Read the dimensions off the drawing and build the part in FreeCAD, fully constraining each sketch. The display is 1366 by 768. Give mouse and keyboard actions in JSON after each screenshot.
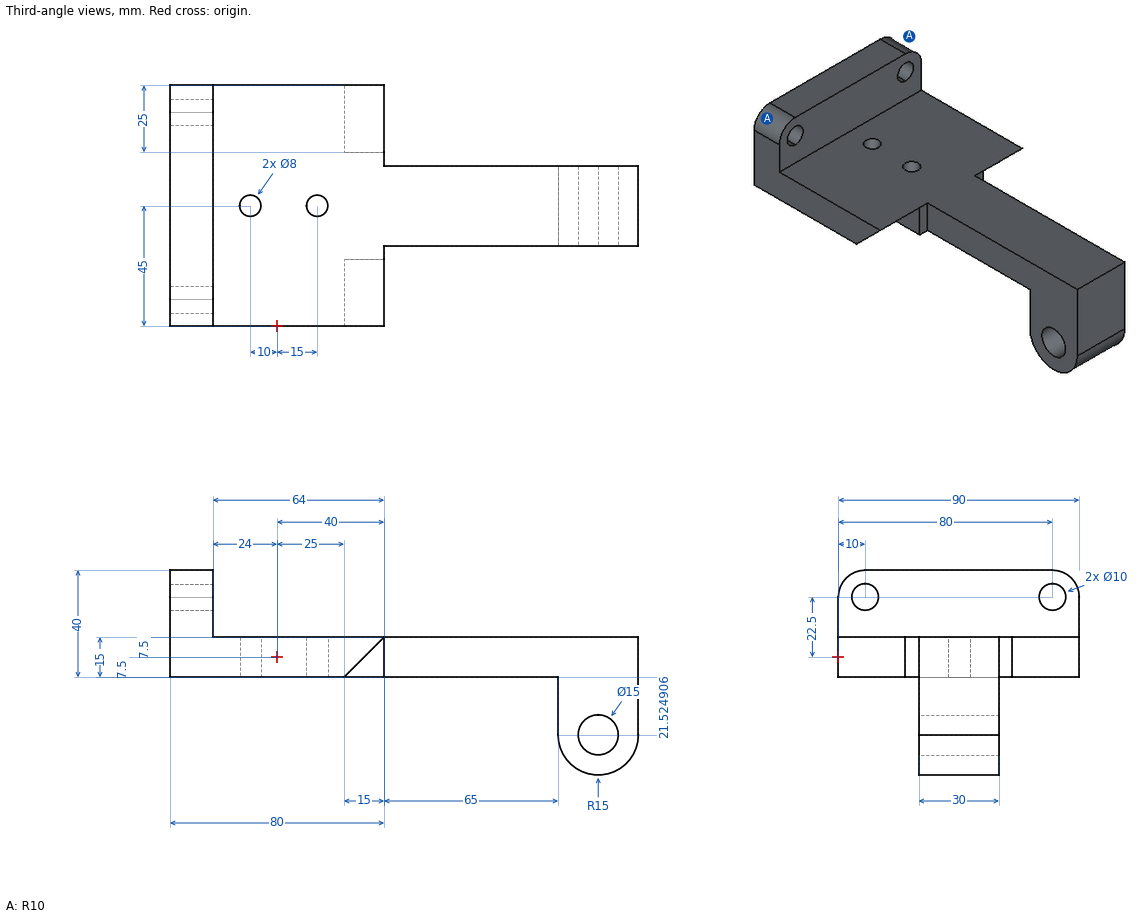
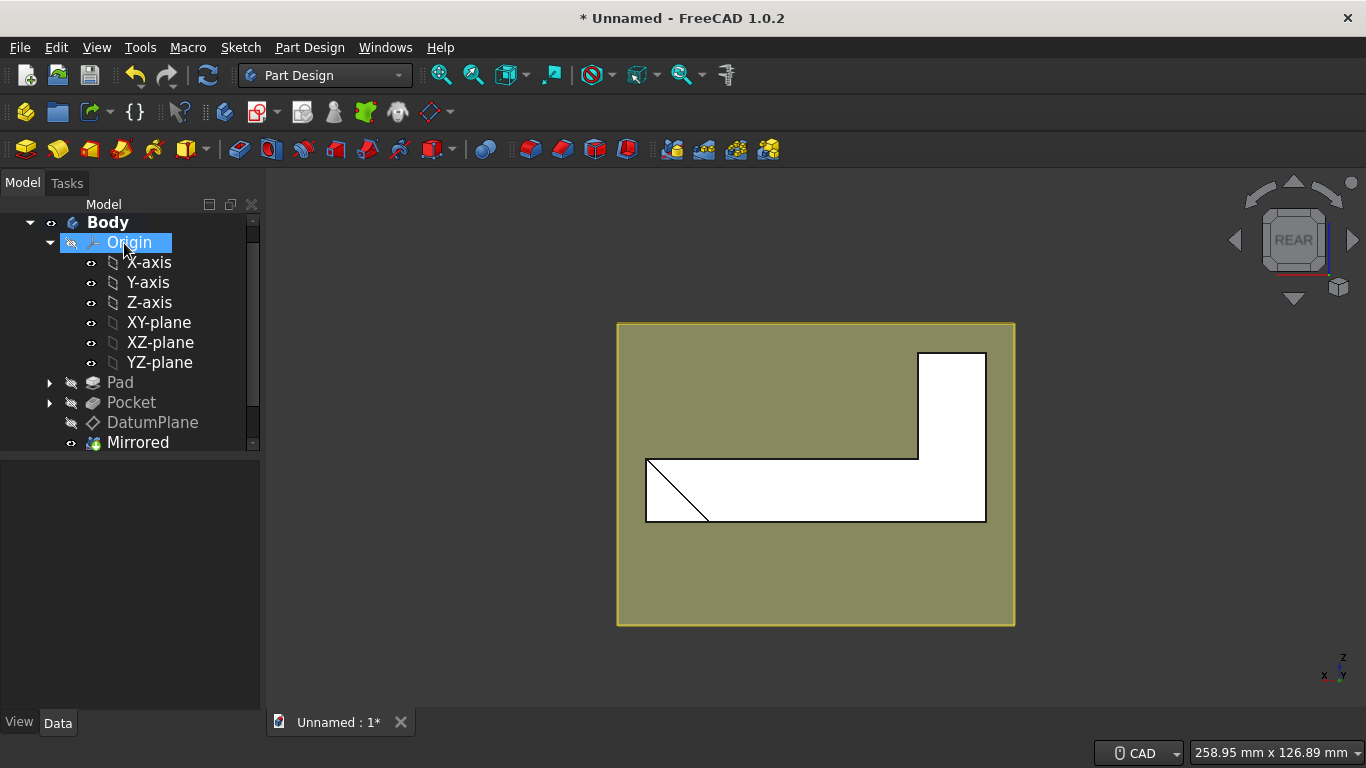
{"action": "scroll", "coordinate": [120, 338], "scroll_direction": "down", "scroll_amount": 3}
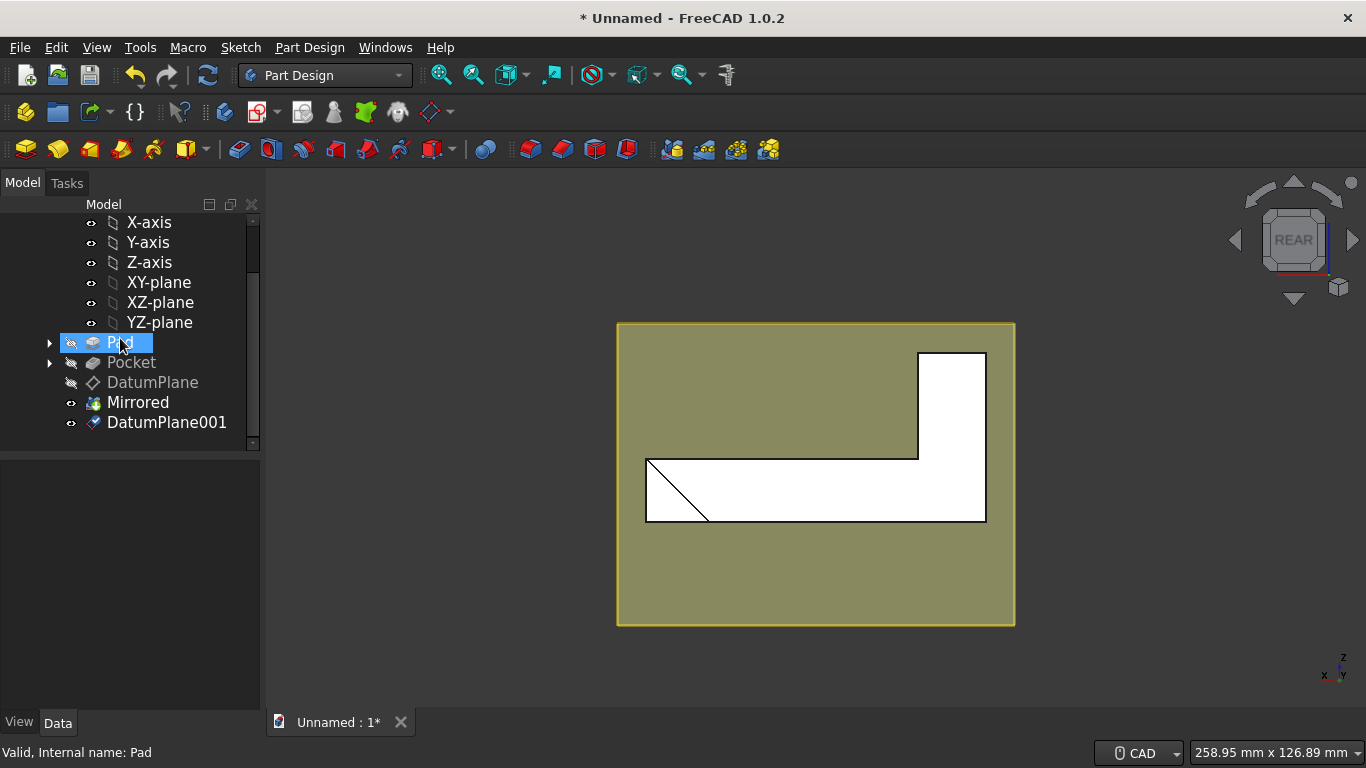
{"action": "left_click", "coordinate": [116, 423]}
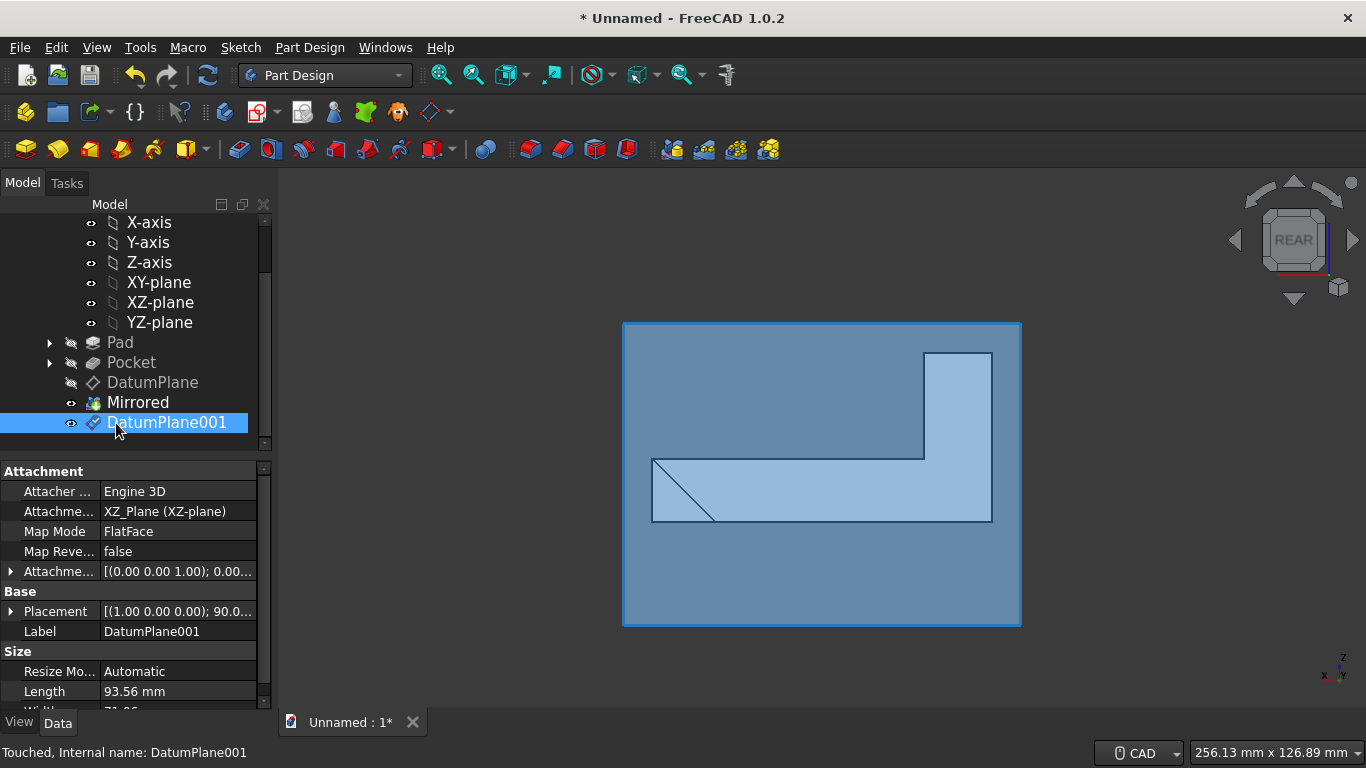
{"action": "left_click", "coordinate": [258, 112]}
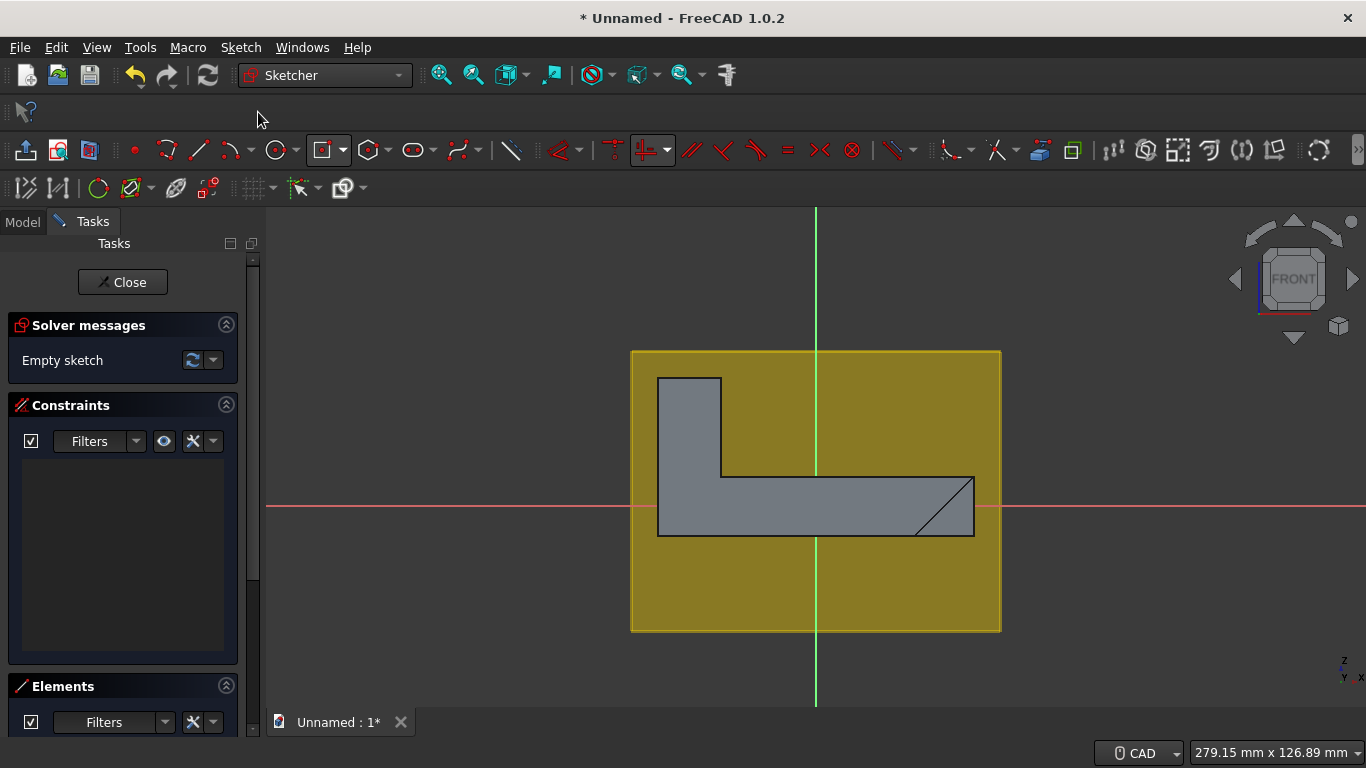
{"action": "left_click", "coordinate": [90, 150]}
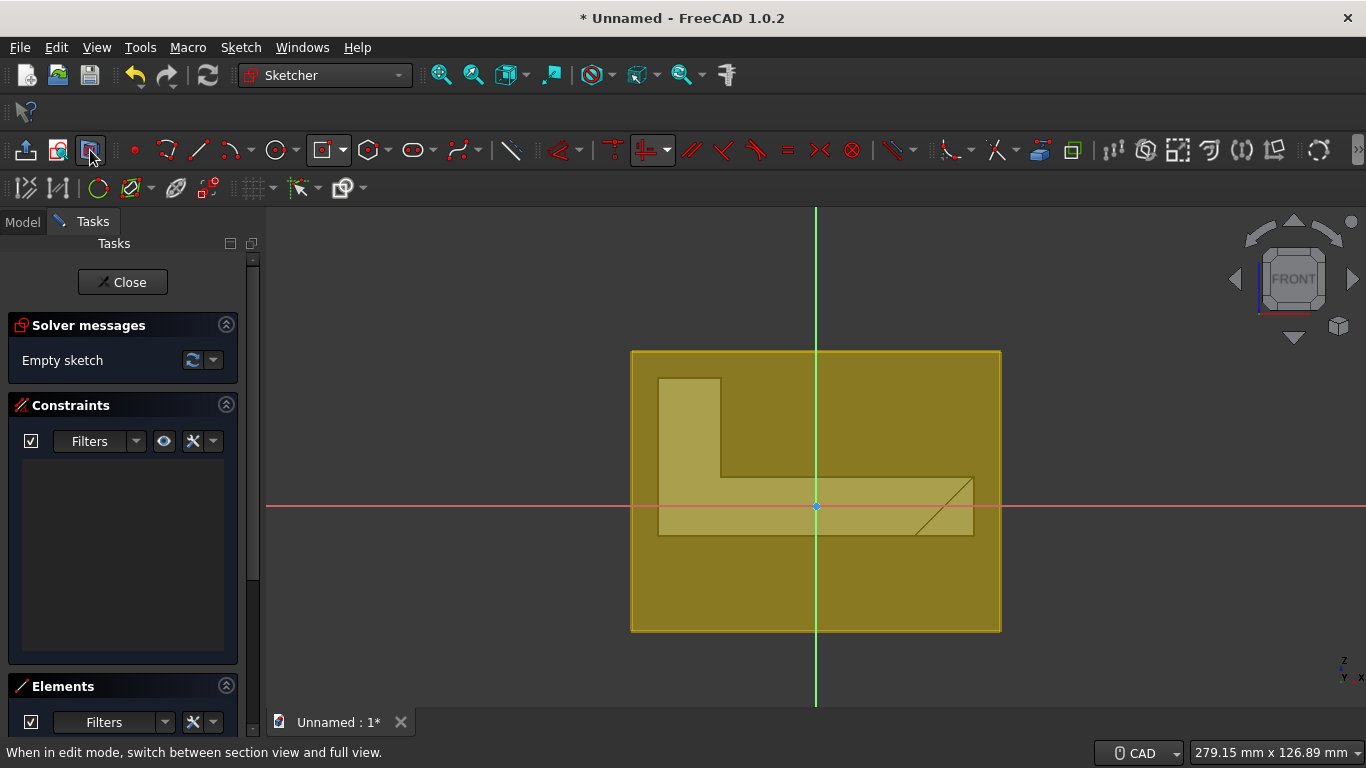
{"action": "scroll", "coordinate": [294, 235], "scroll_direction": "down", "scroll_amount": 1}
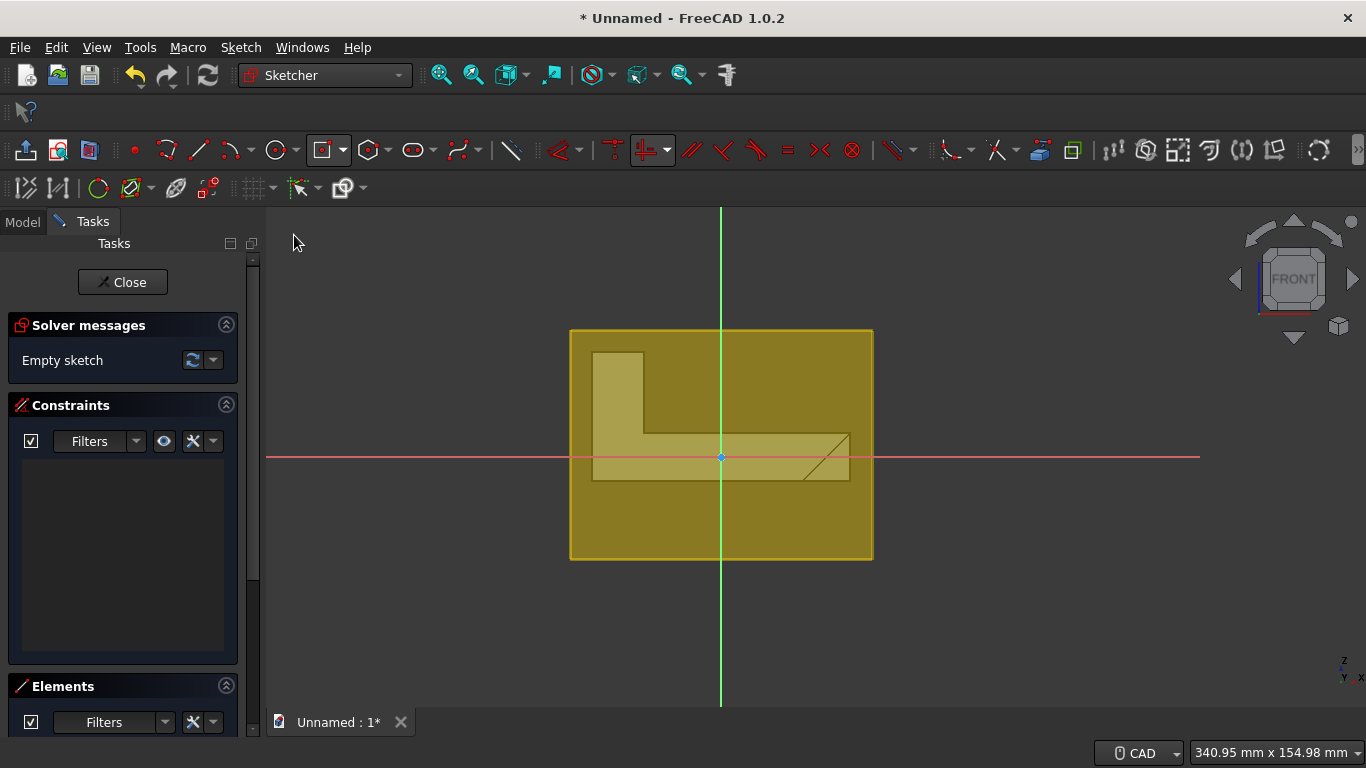
{"action": "scroll", "coordinate": [1201, 636], "scroll_direction": "up", "scroll_amount": 2}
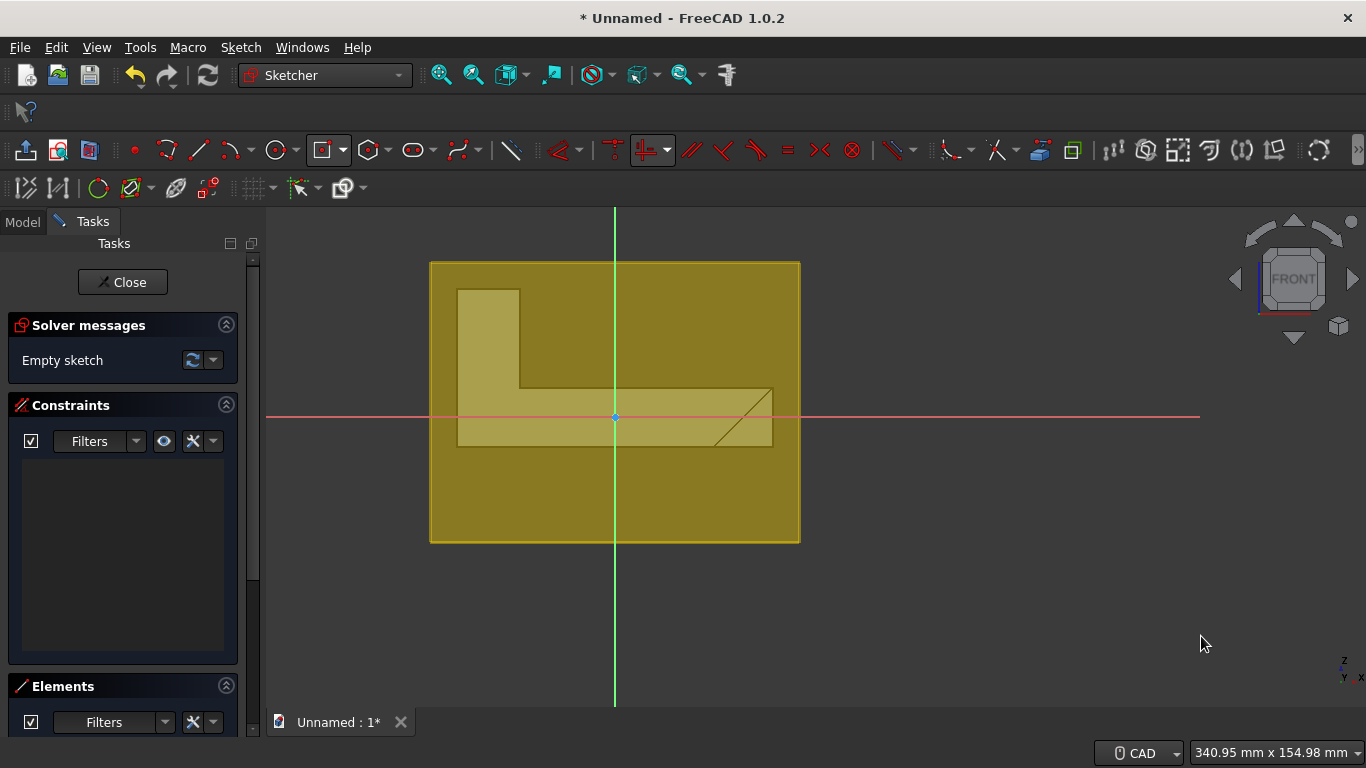
{"action": "left_click", "coordinate": [168, 150]}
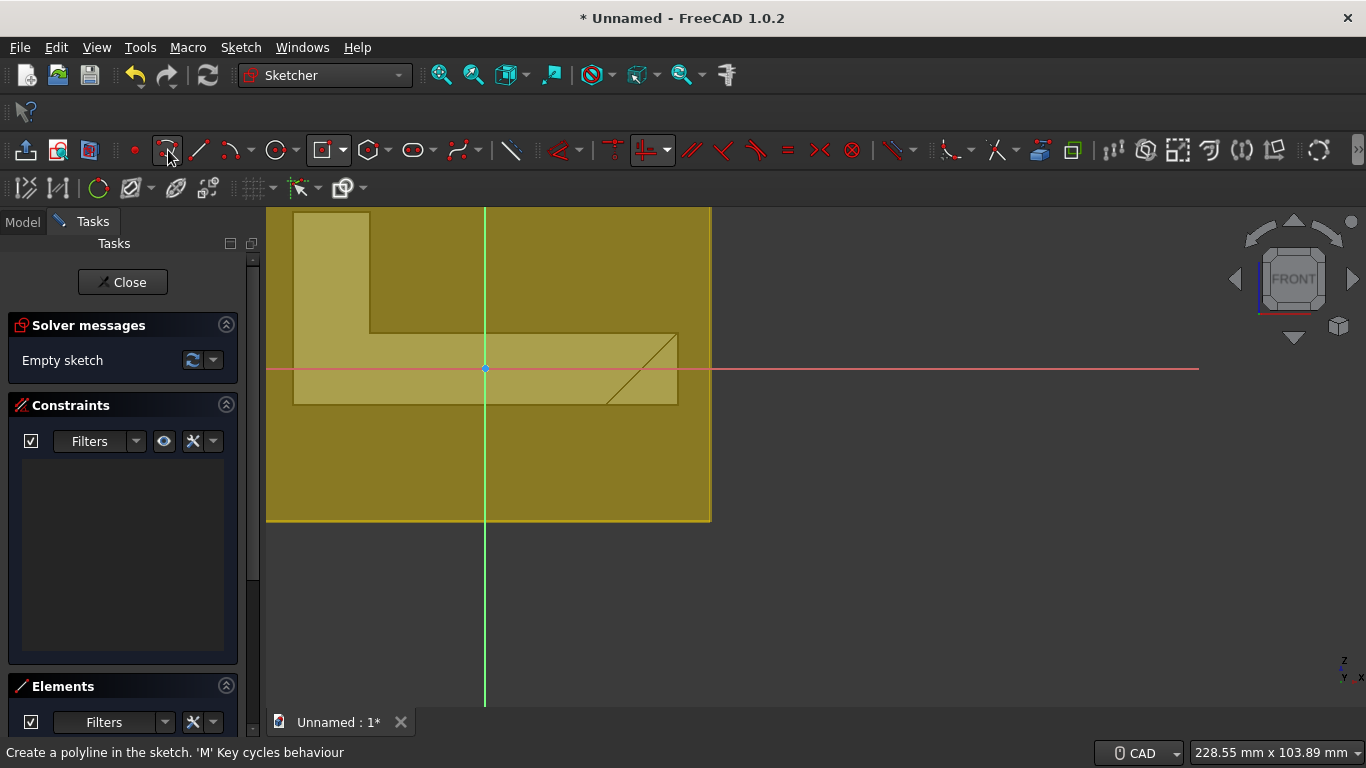
{"action": "left_click", "coordinate": [990, 508]}
{"action": "left_click", "coordinate": [990, 405]}
{"action": "left_click", "coordinate": [678, 405]}
{"action": "left_click", "coordinate": [678, 333]}
{"action": "left_click", "coordinate": [1135, 333]}
{"action": "left_click", "coordinate": [1135, 508]}
{"action": "right_click", "coordinate": [1135, 508]}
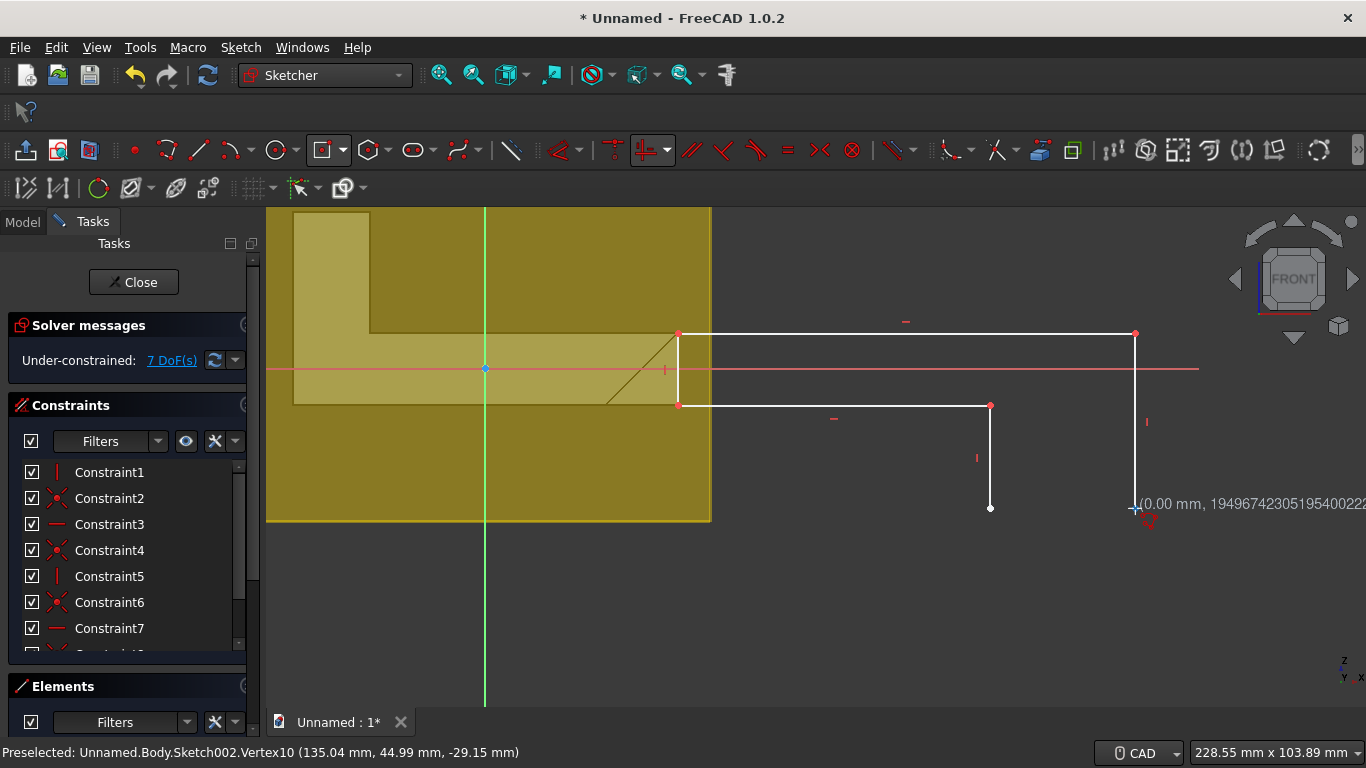
{"action": "left_click", "coordinate": [254, 150]}